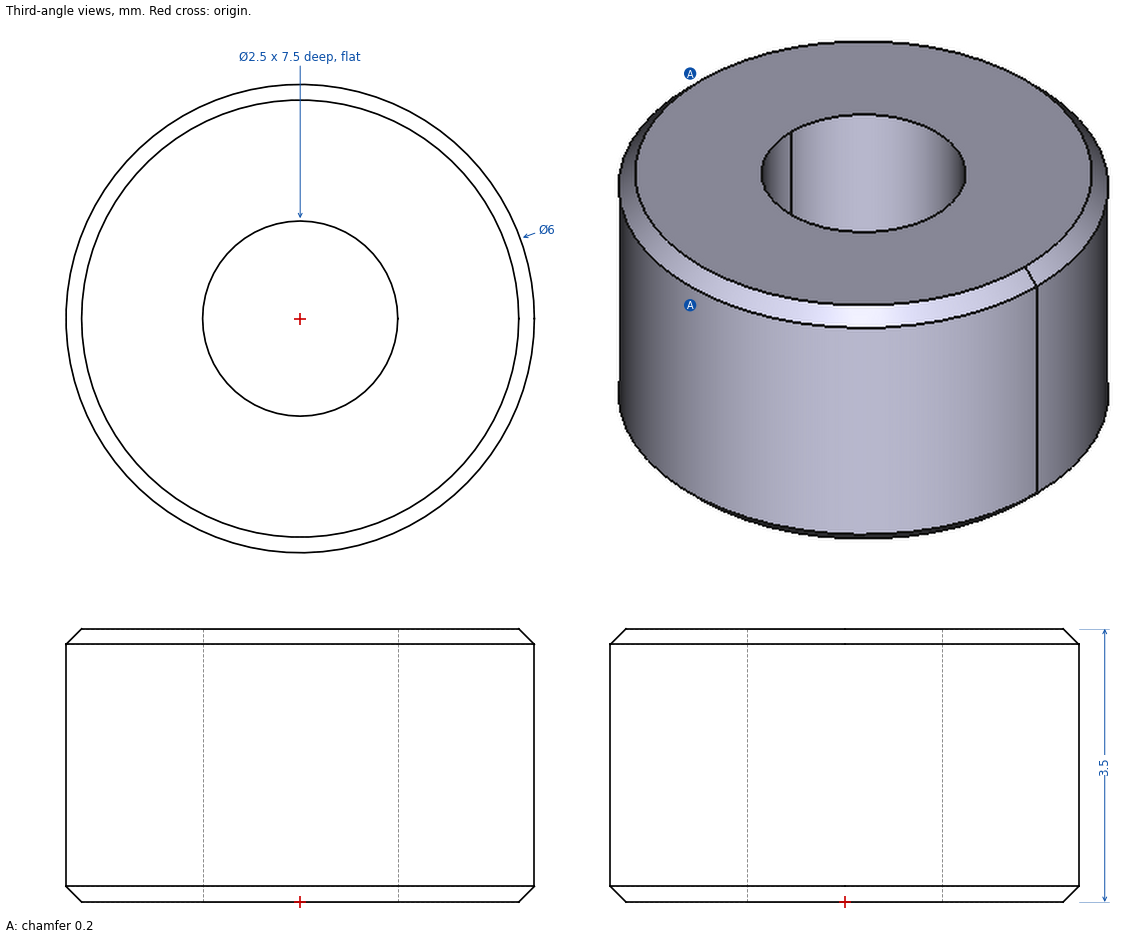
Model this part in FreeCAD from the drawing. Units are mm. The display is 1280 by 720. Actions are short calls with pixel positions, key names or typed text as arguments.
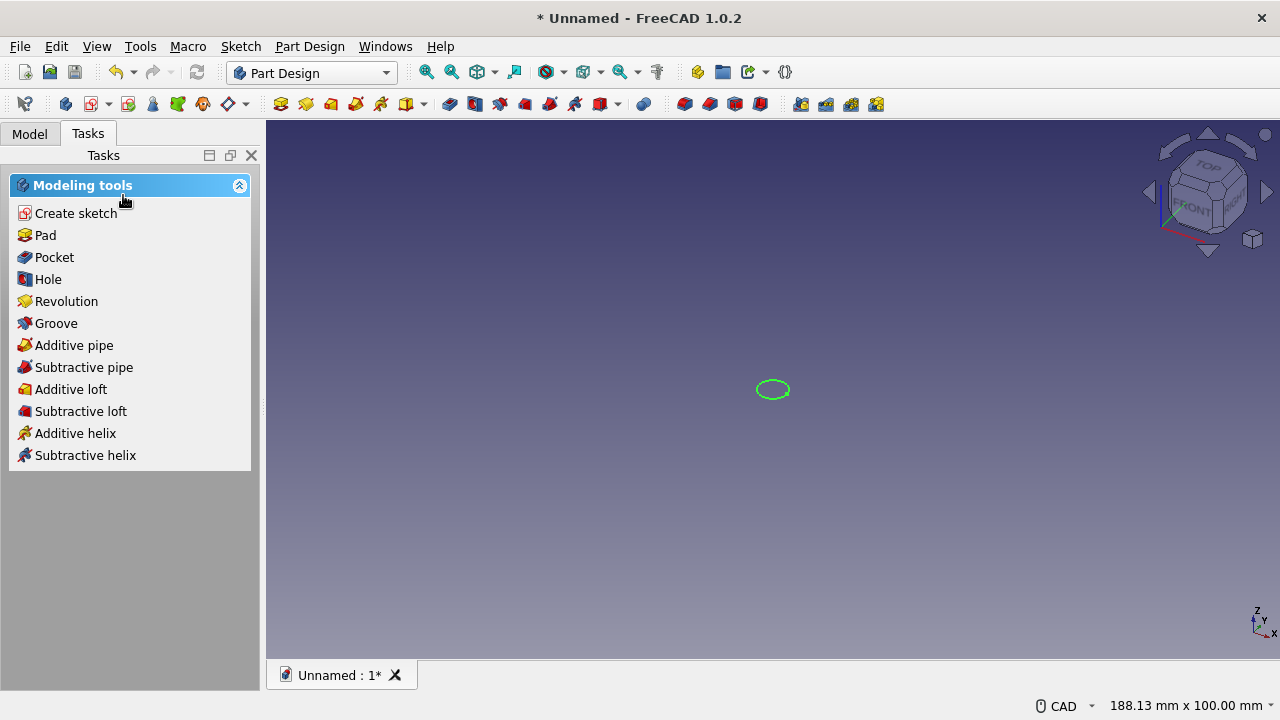
click(281, 104)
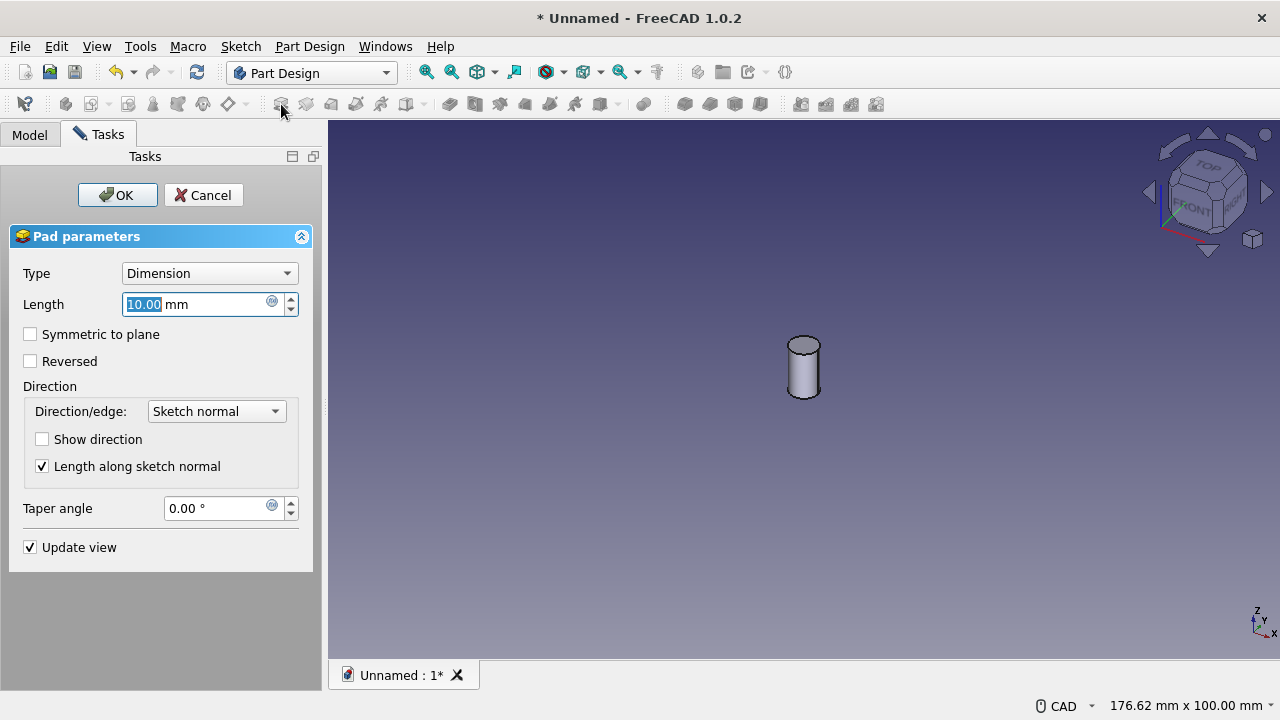
text(3.5)
key(Tab)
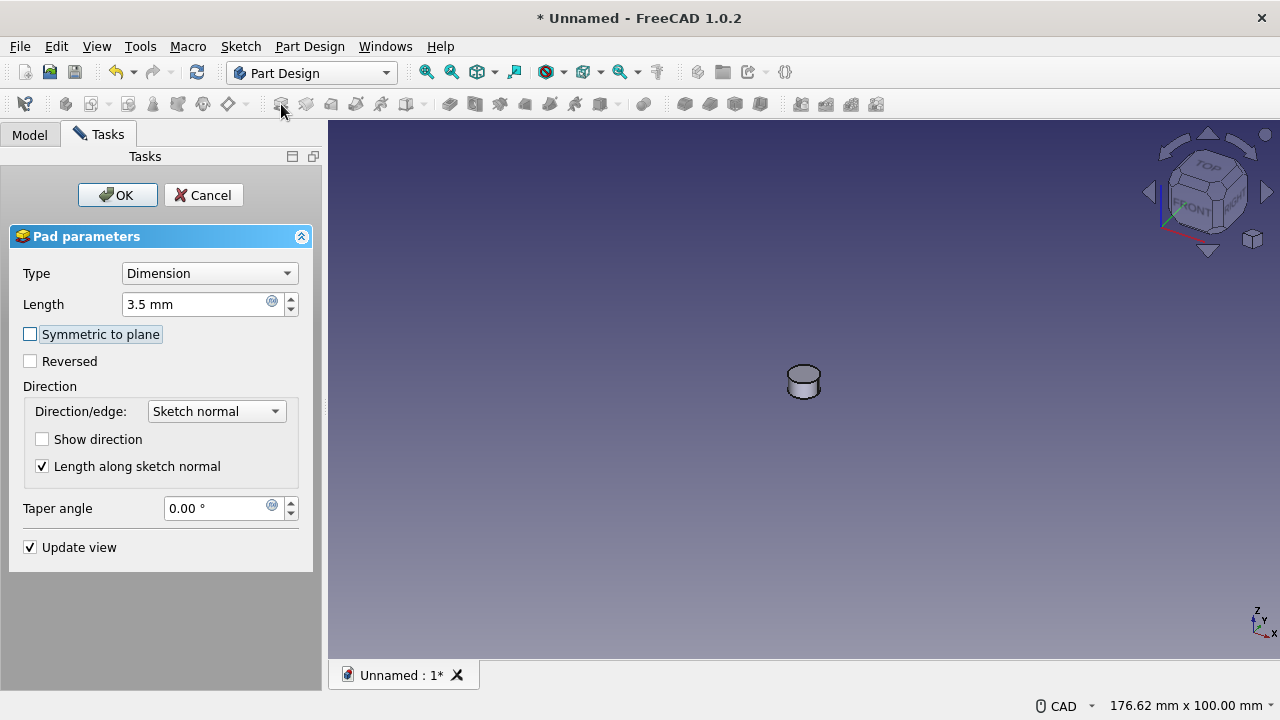
click(118, 195)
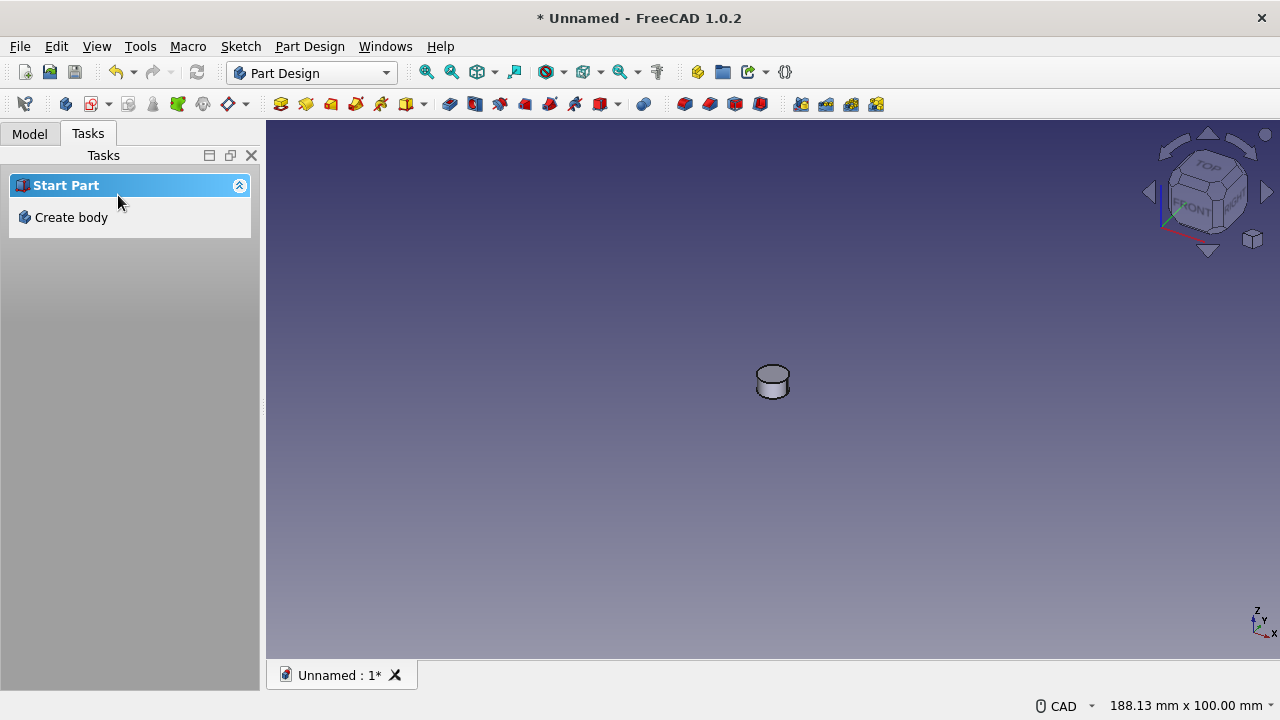
key(v)
key(f)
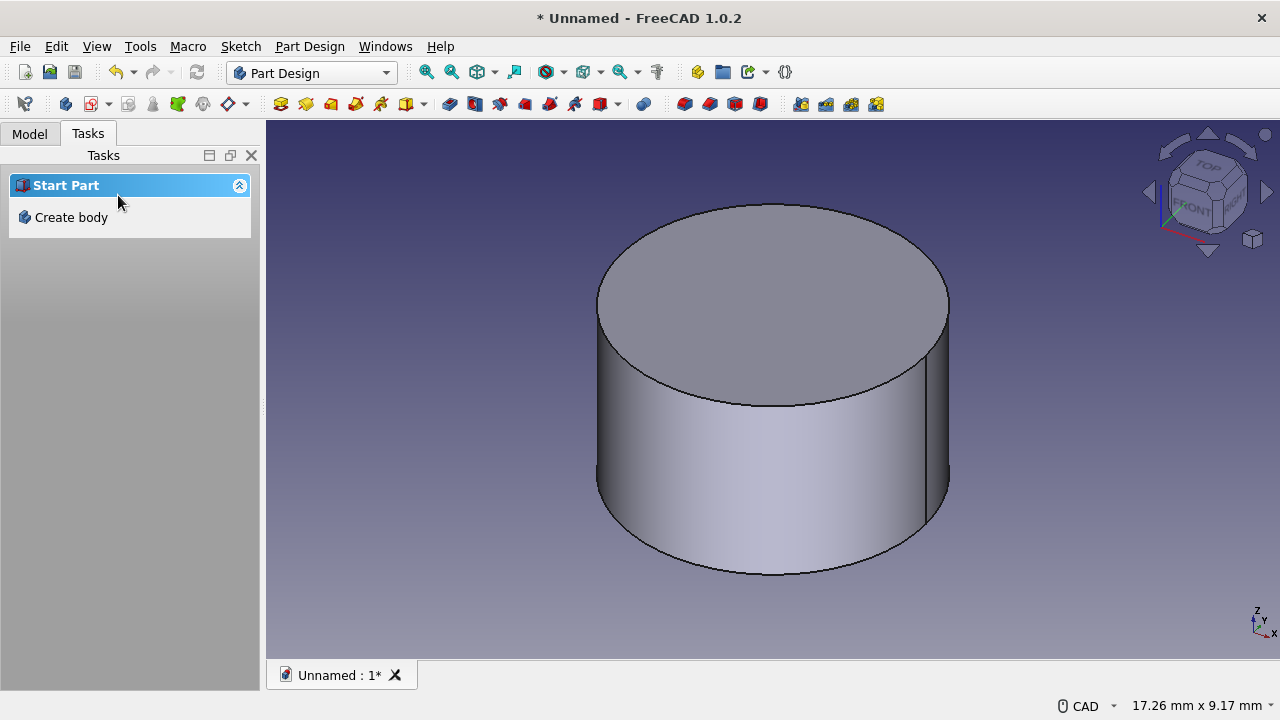
click(90, 104)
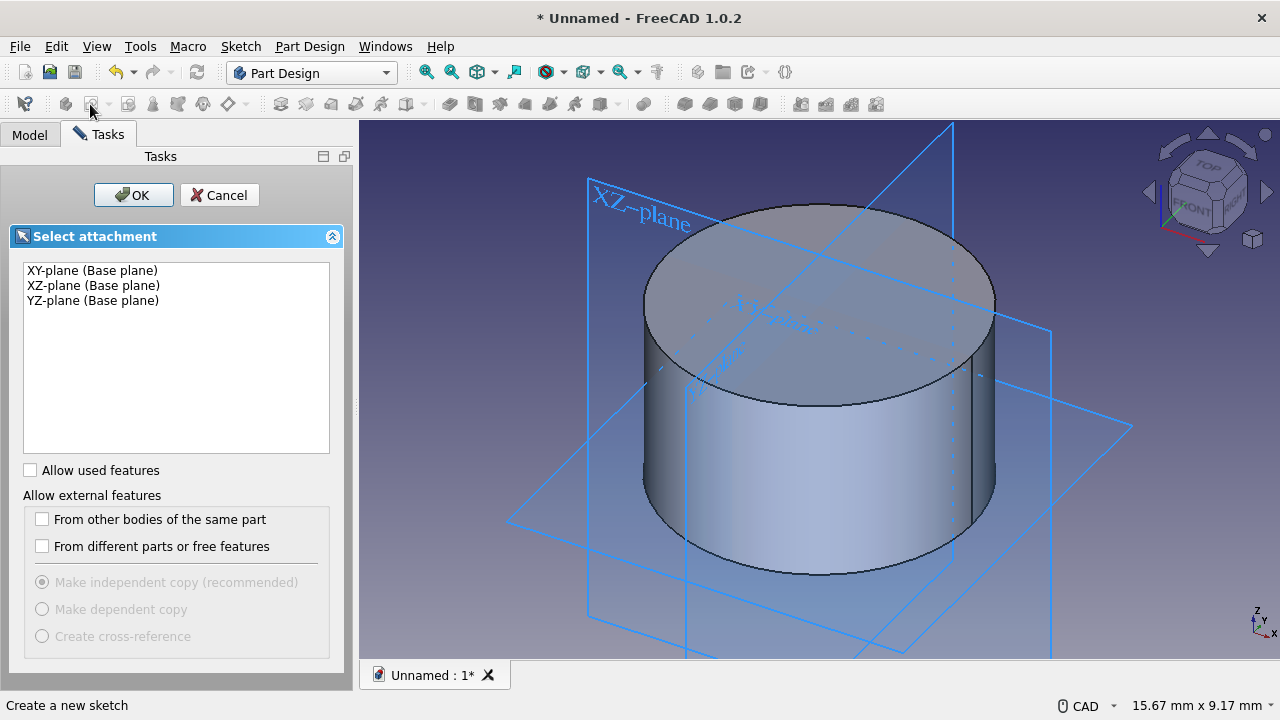
click(84, 270)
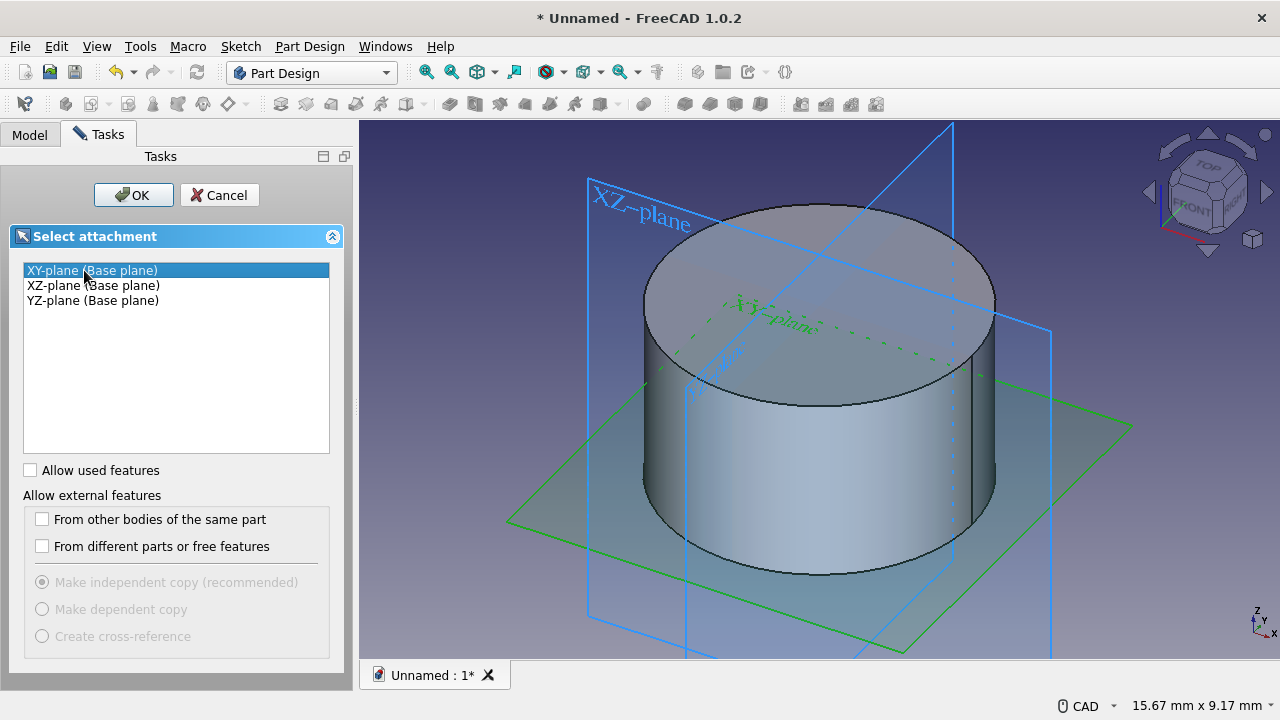
click(134, 195)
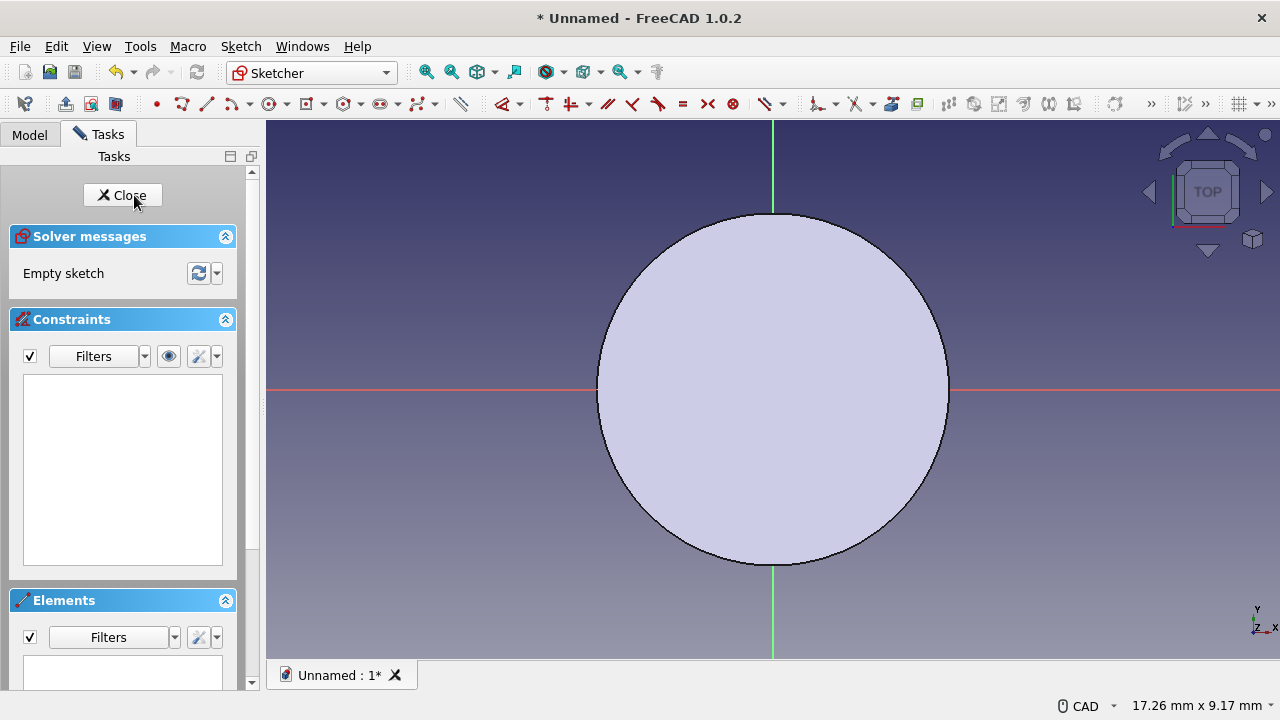
key(q)
key(s)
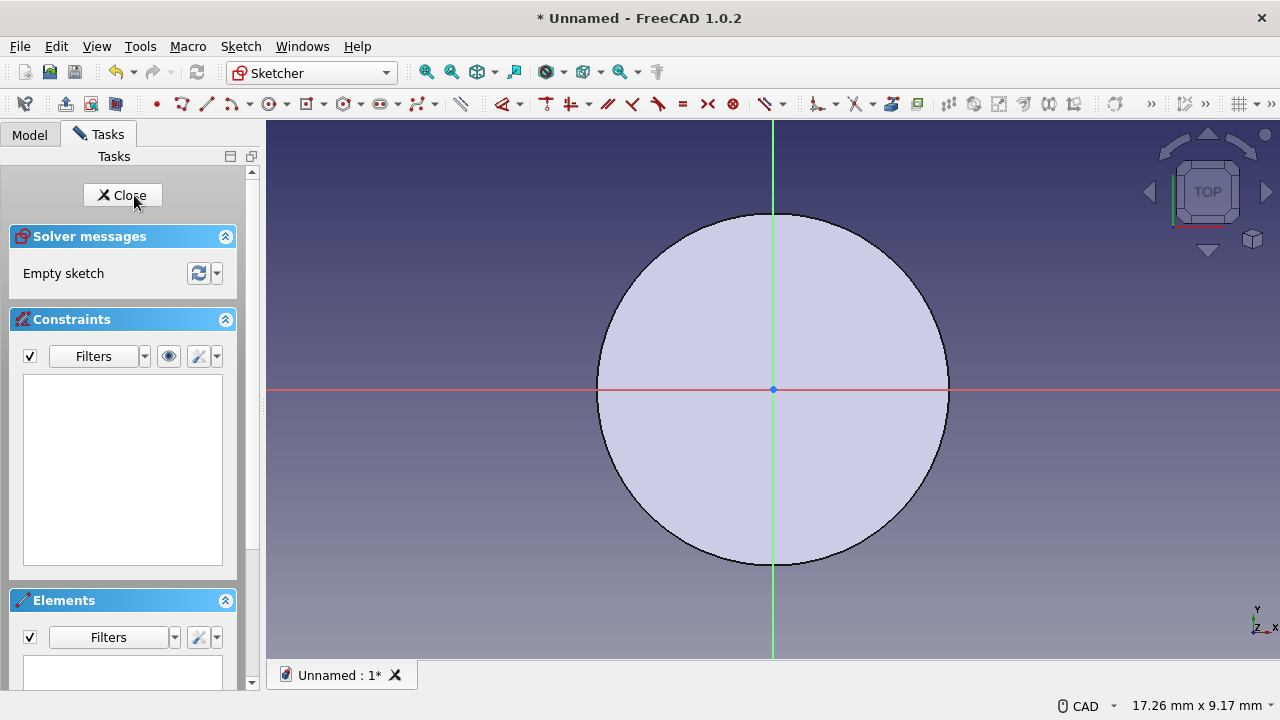
scroll(829, 390, up, 4)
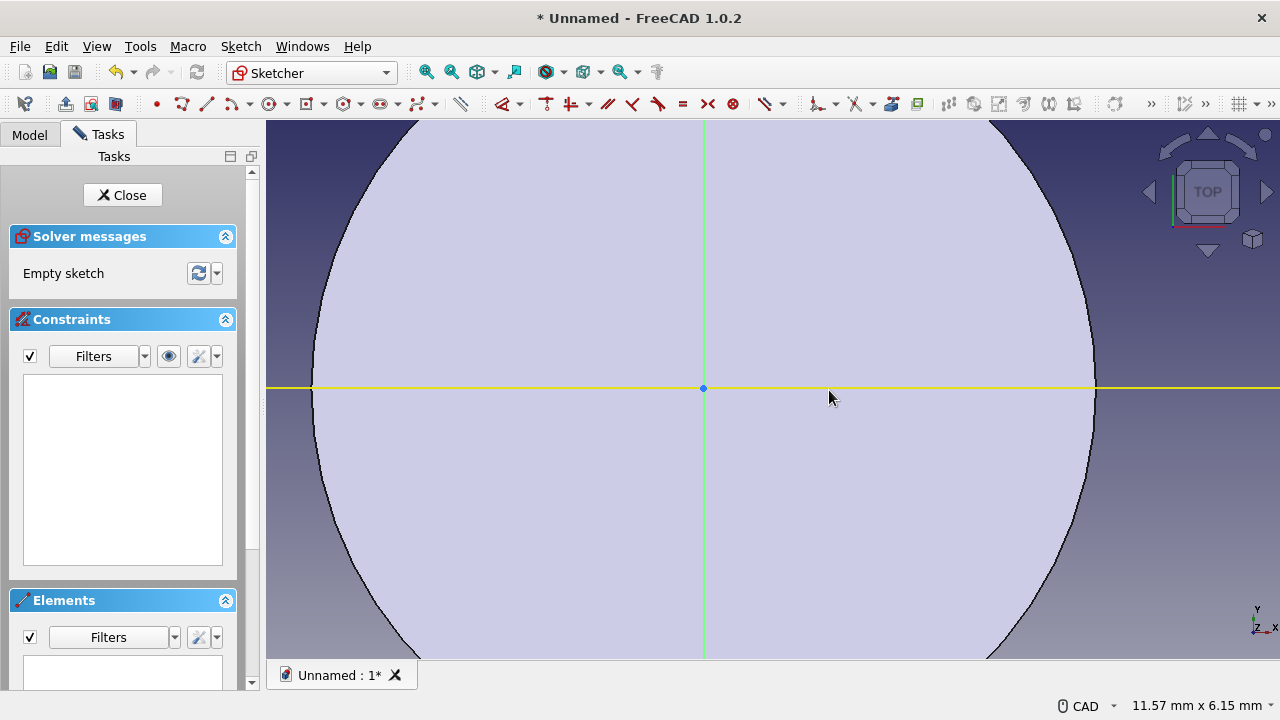
key(g)
key(c)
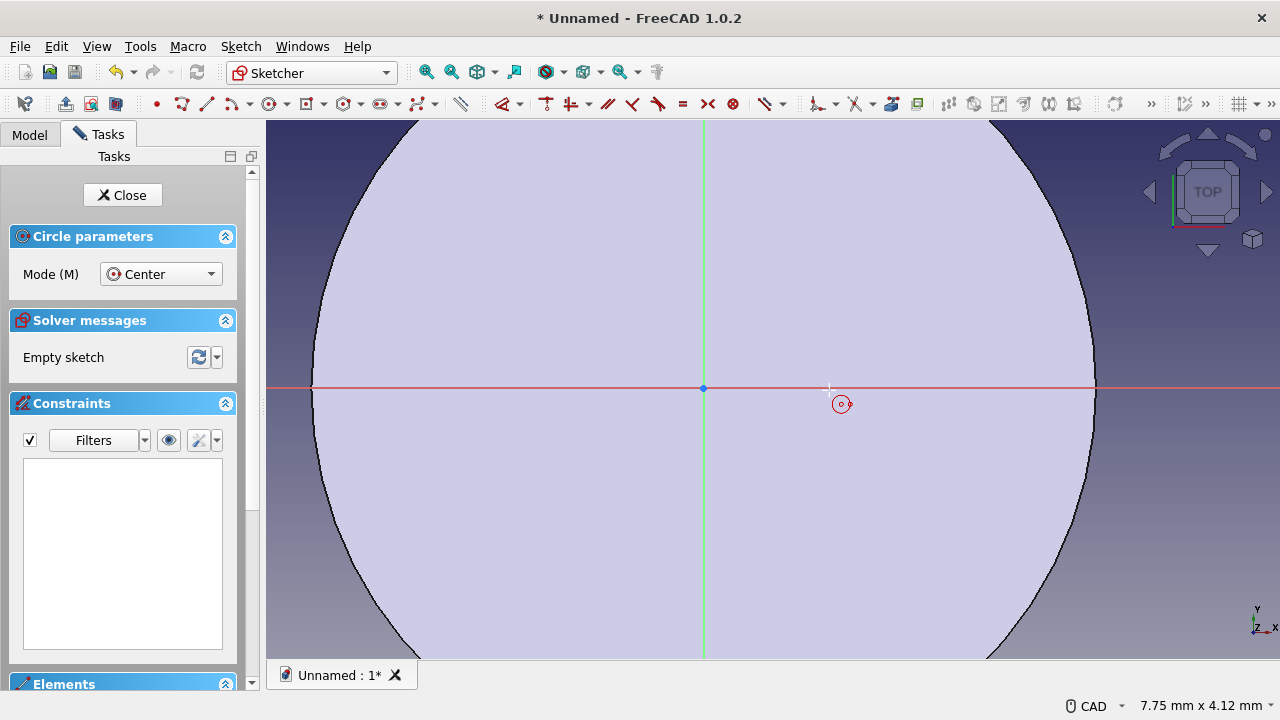
click(704, 388)
click(819, 273)
key(Escape)